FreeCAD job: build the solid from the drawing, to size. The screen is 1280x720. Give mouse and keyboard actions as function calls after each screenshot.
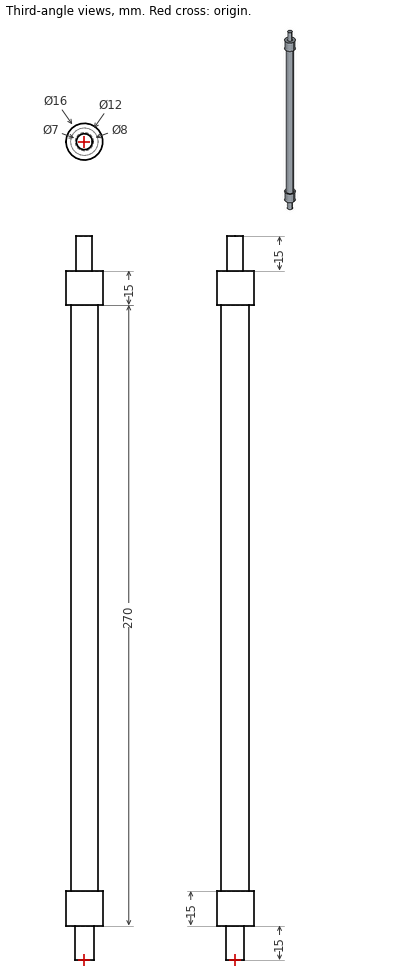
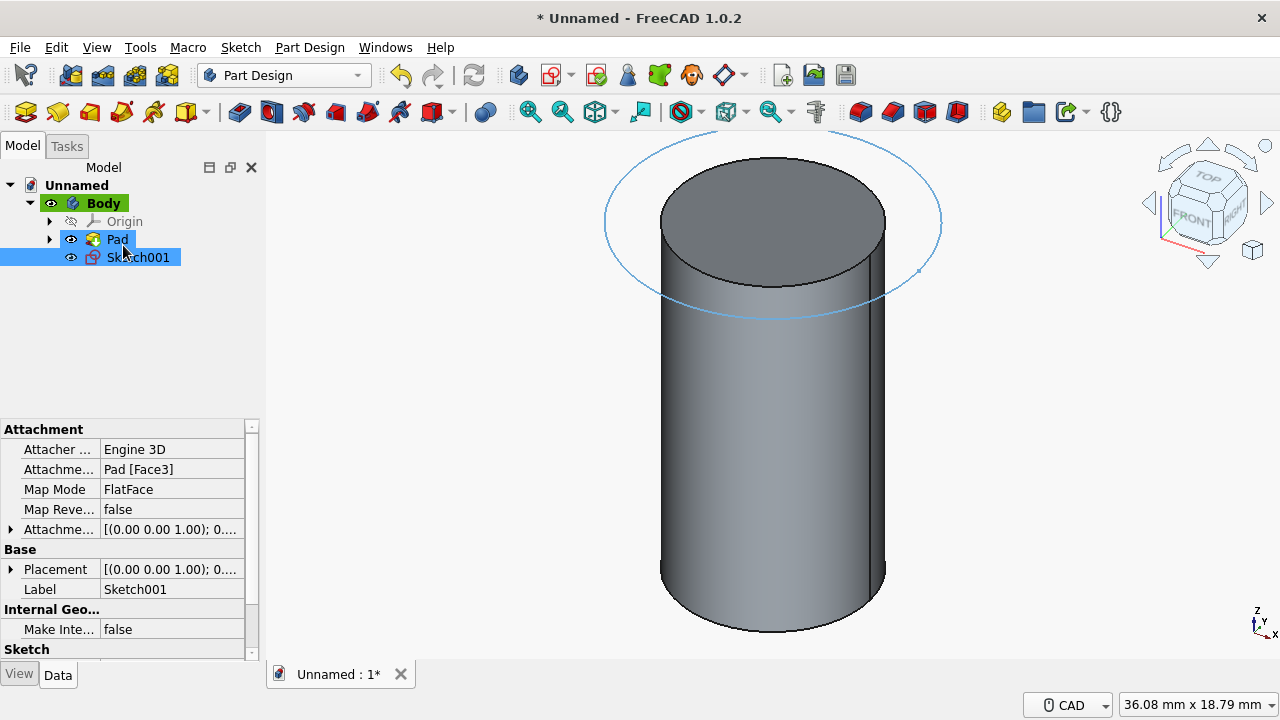
click(26, 112)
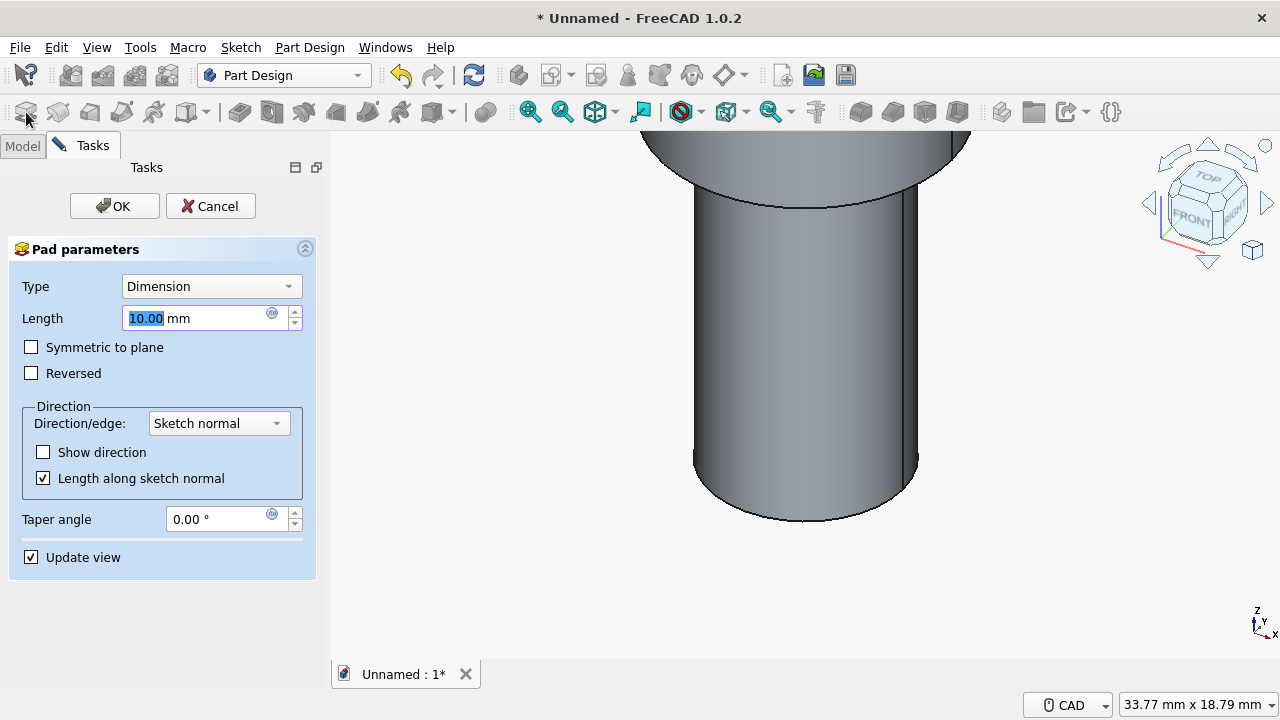
text(270)
key(Tab)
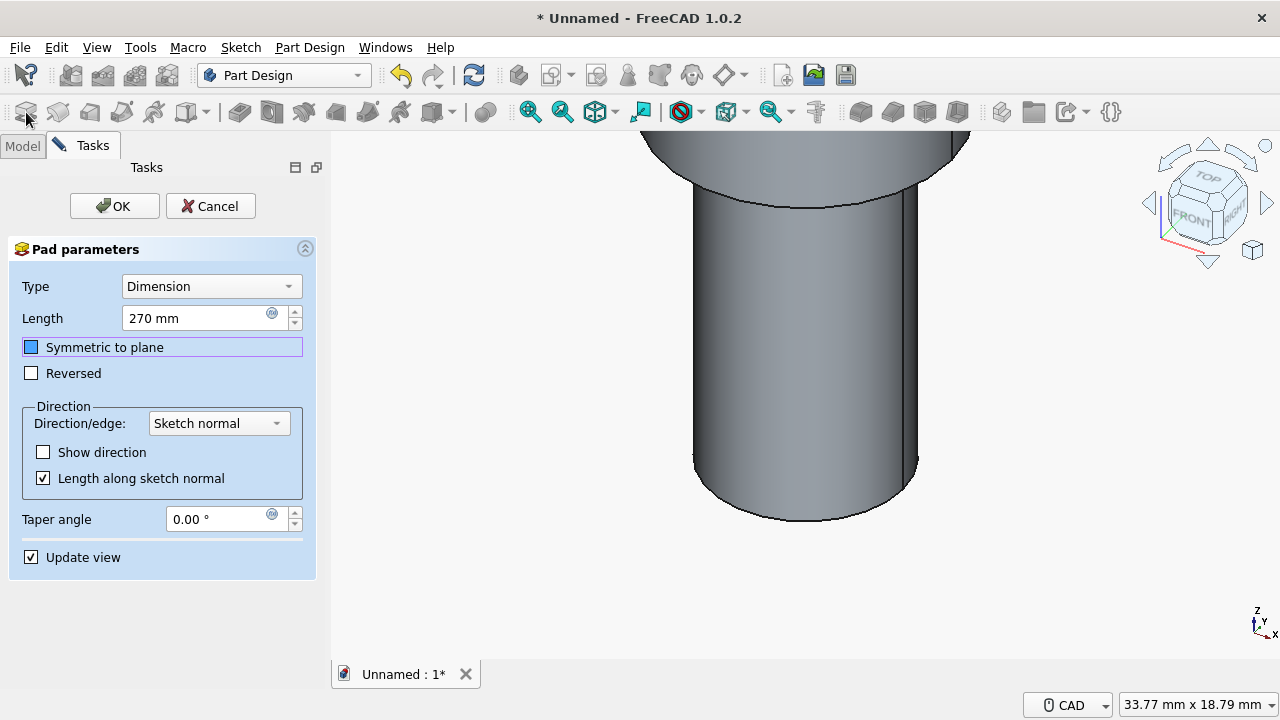
click(115, 206)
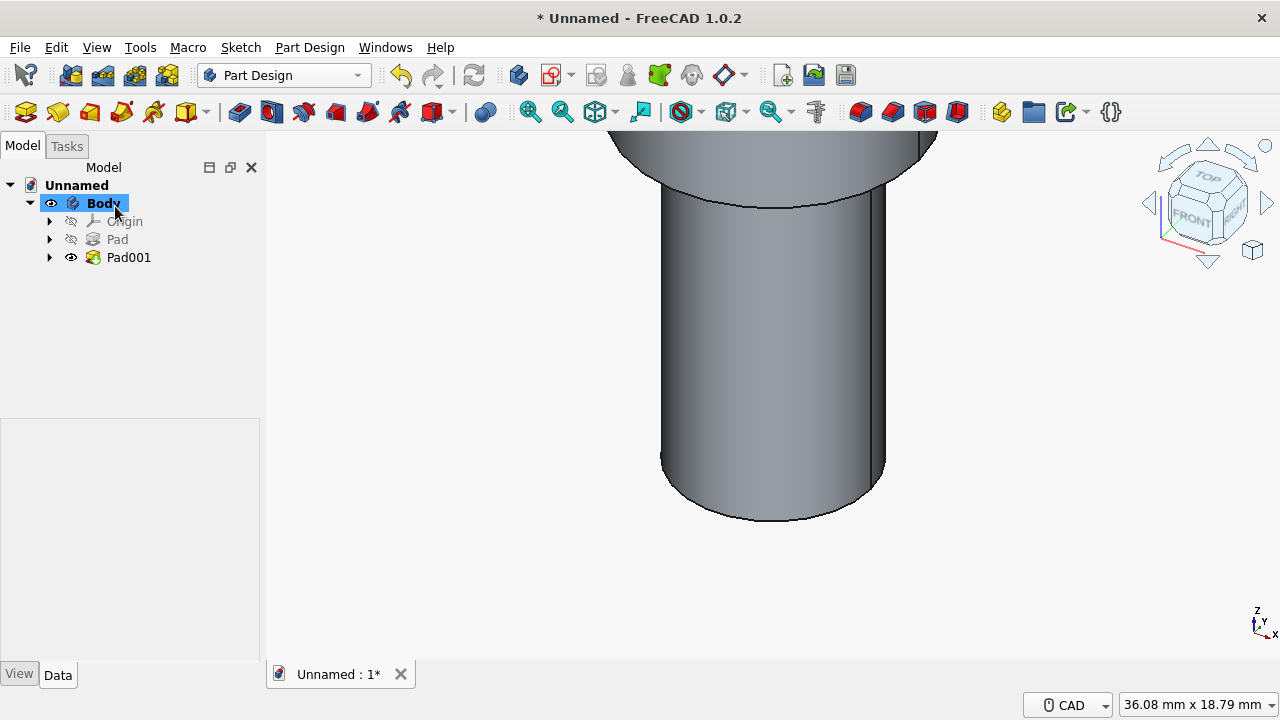
click(532, 112)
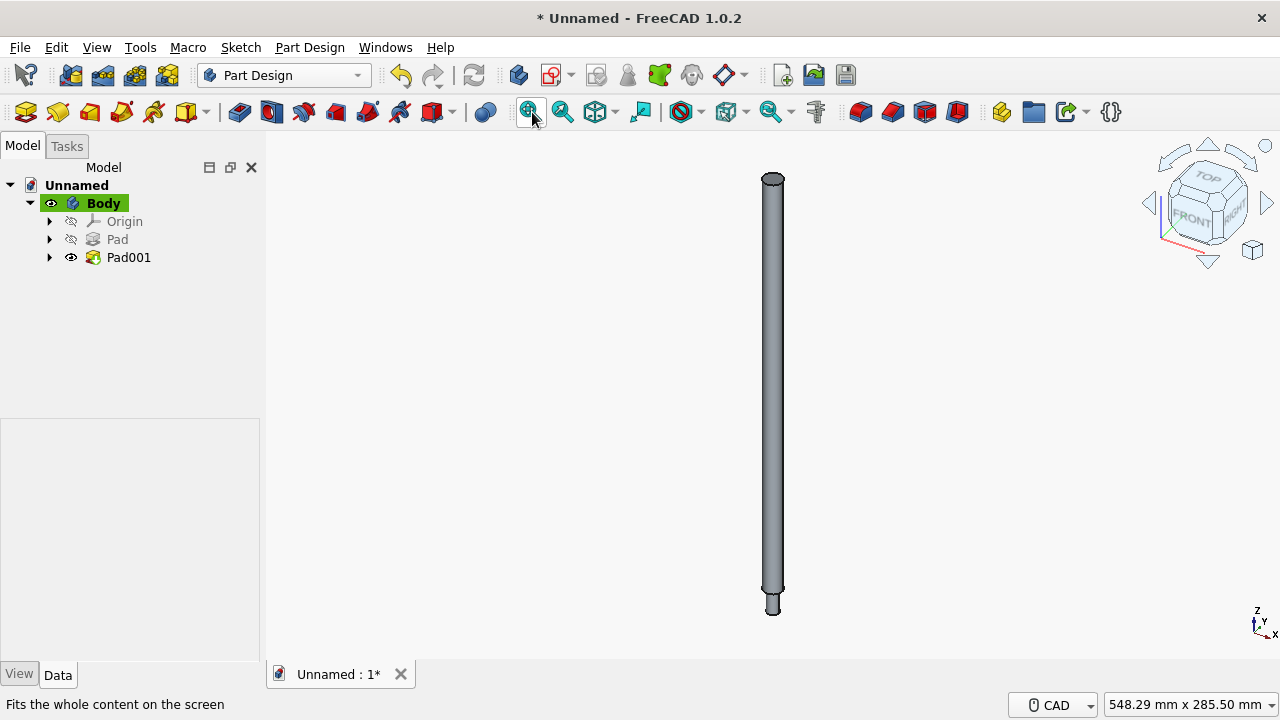
key(5)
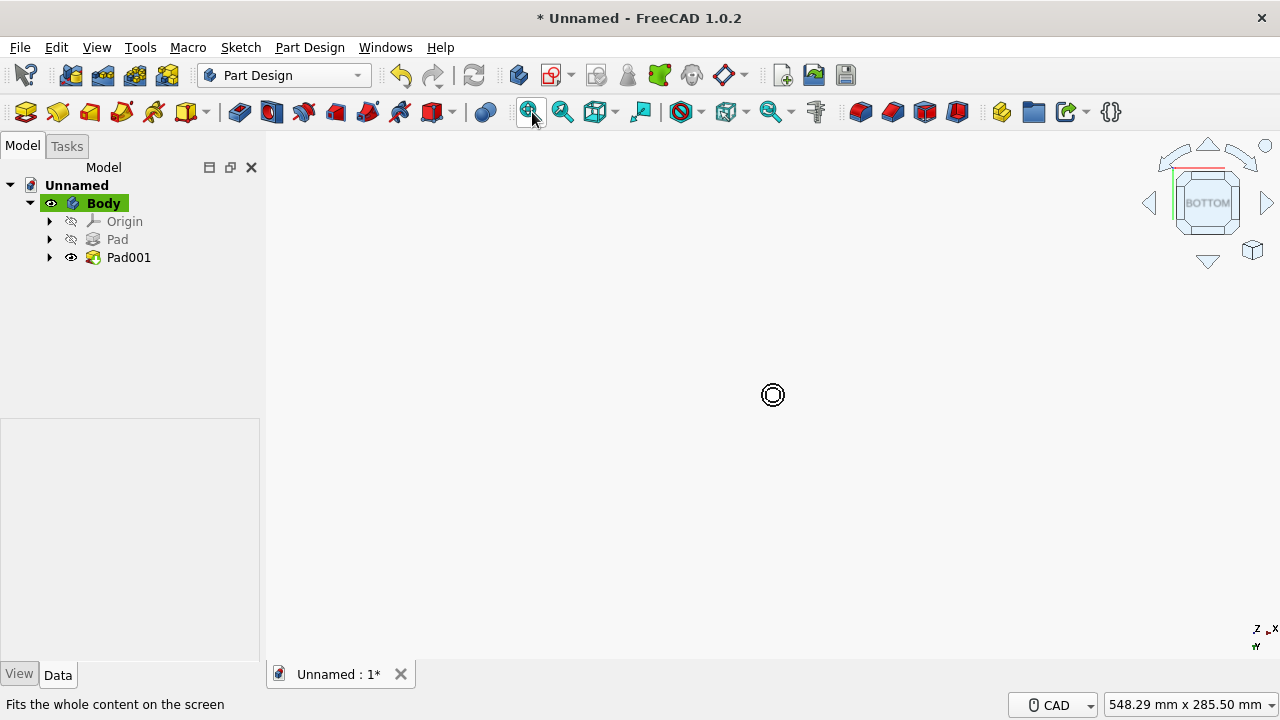
click(532, 112)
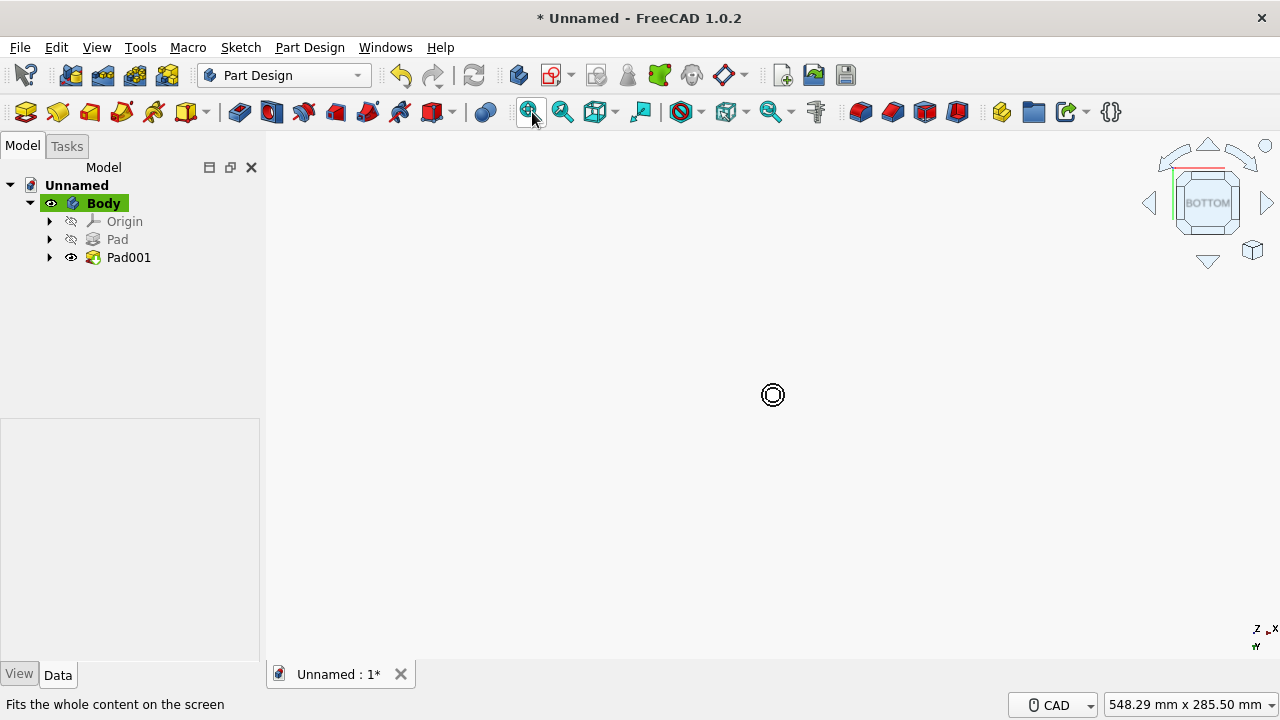
scroll(783, 394, up, 11)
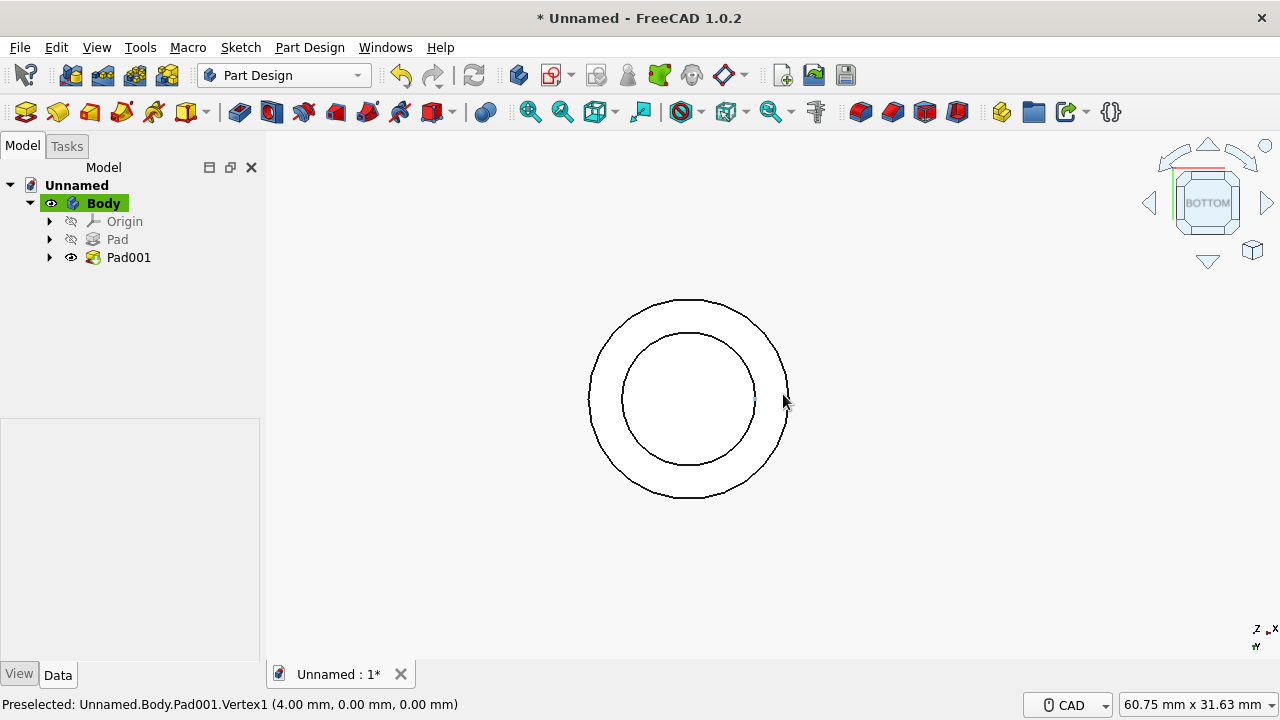
click(774, 398)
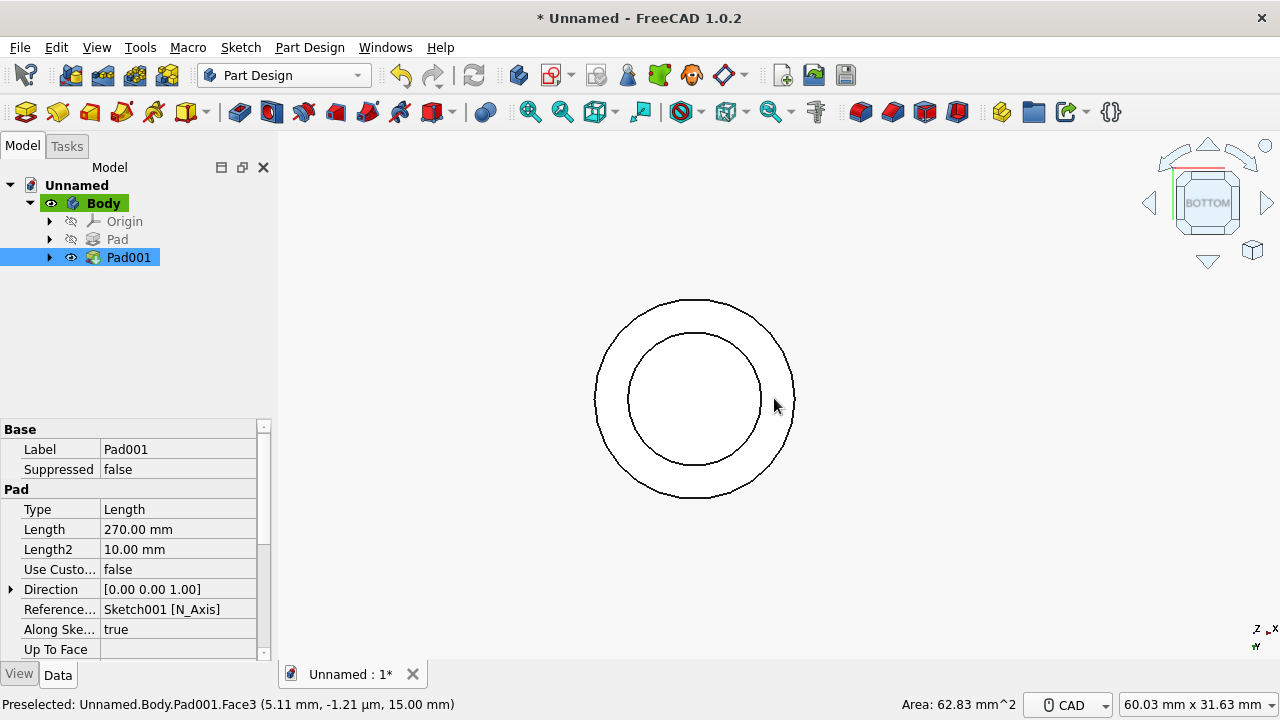
click(552, 76)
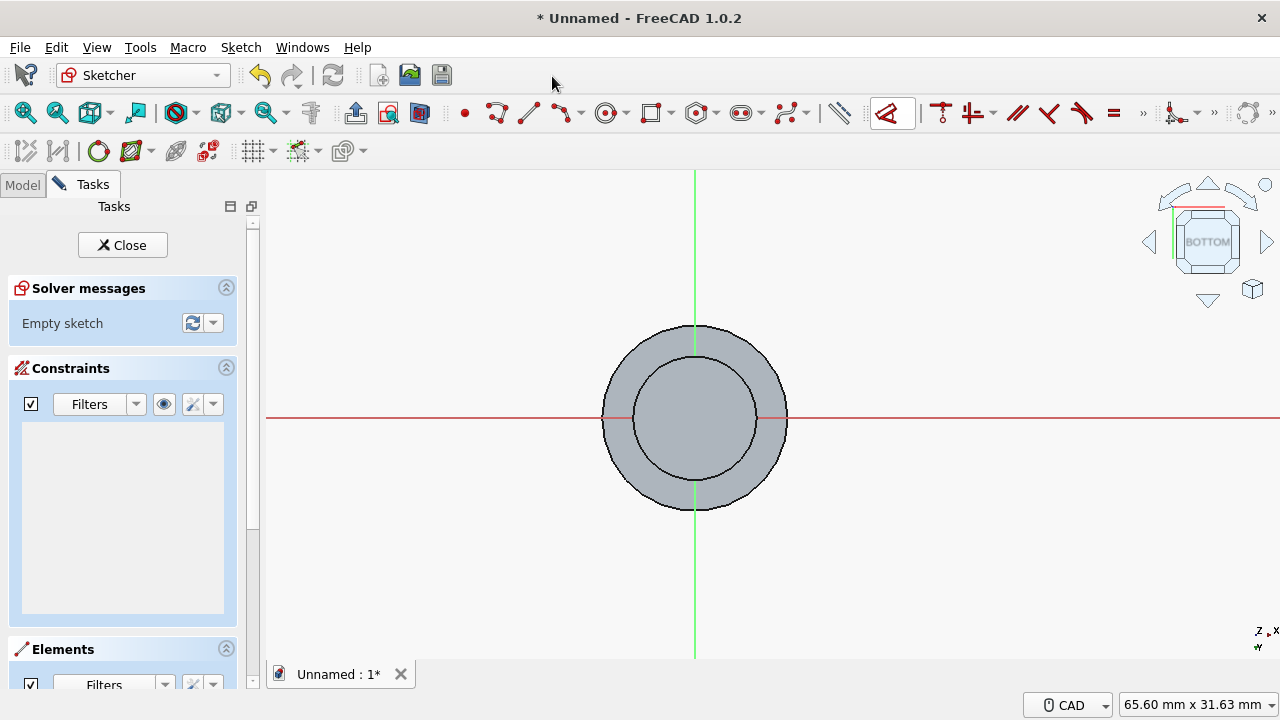
click(420, 114)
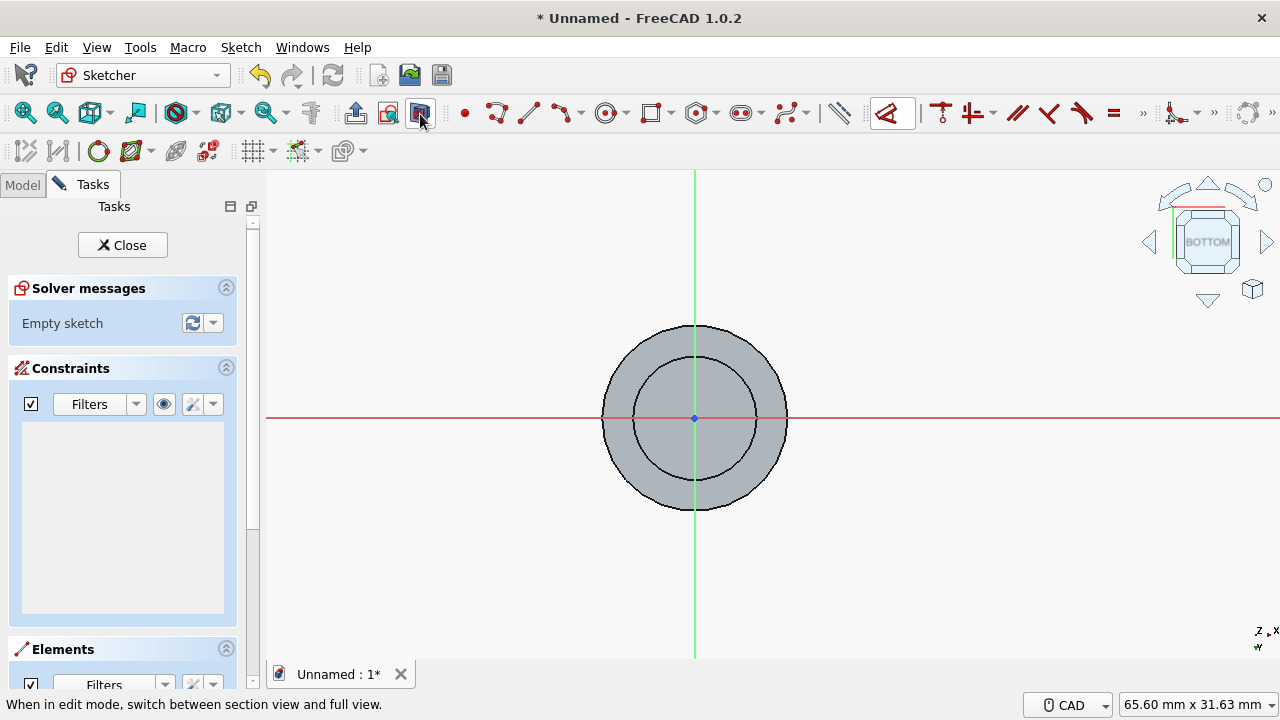
click(606, 114)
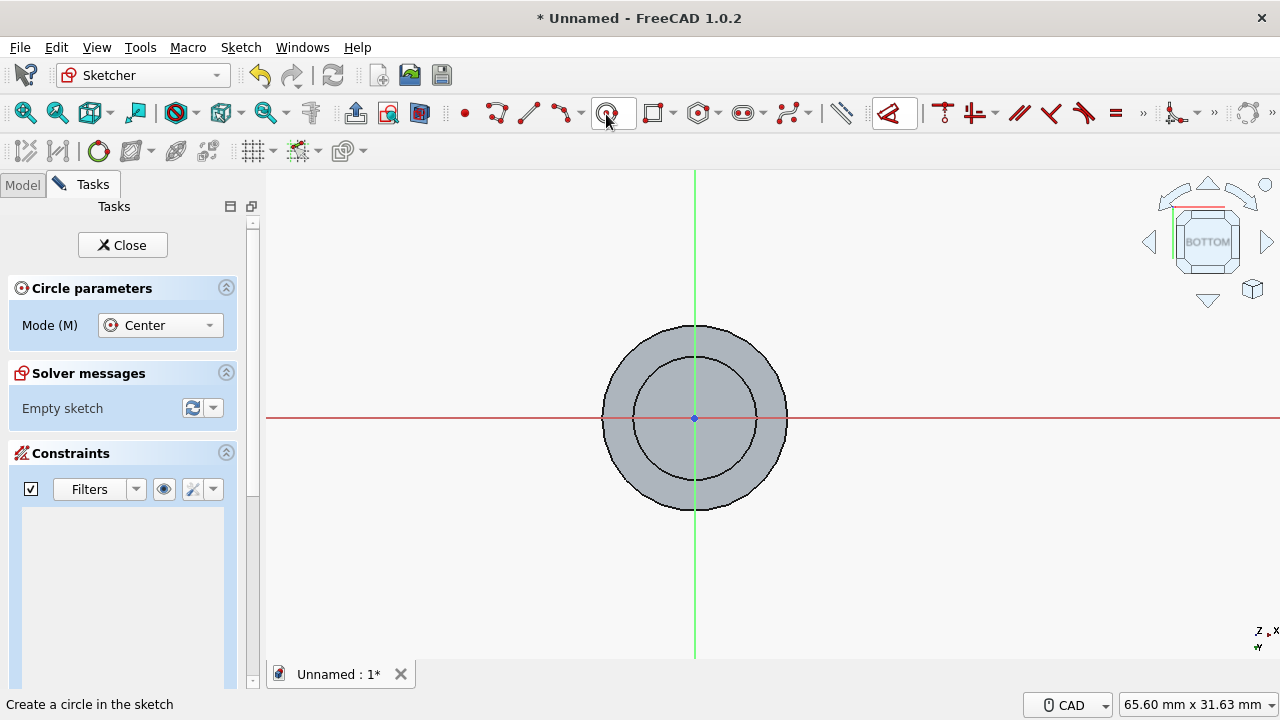
click(695, 418)
click(782, 331)
key(Escape)